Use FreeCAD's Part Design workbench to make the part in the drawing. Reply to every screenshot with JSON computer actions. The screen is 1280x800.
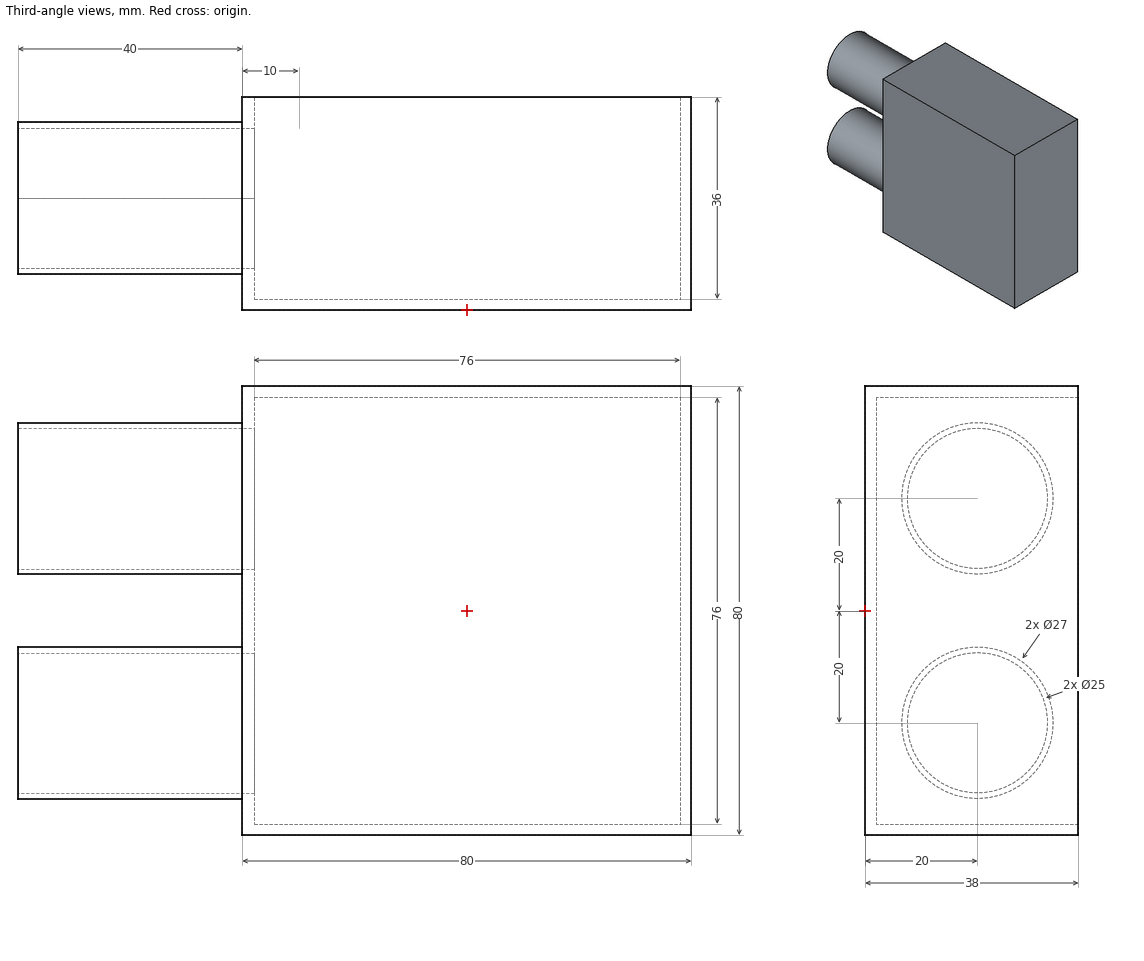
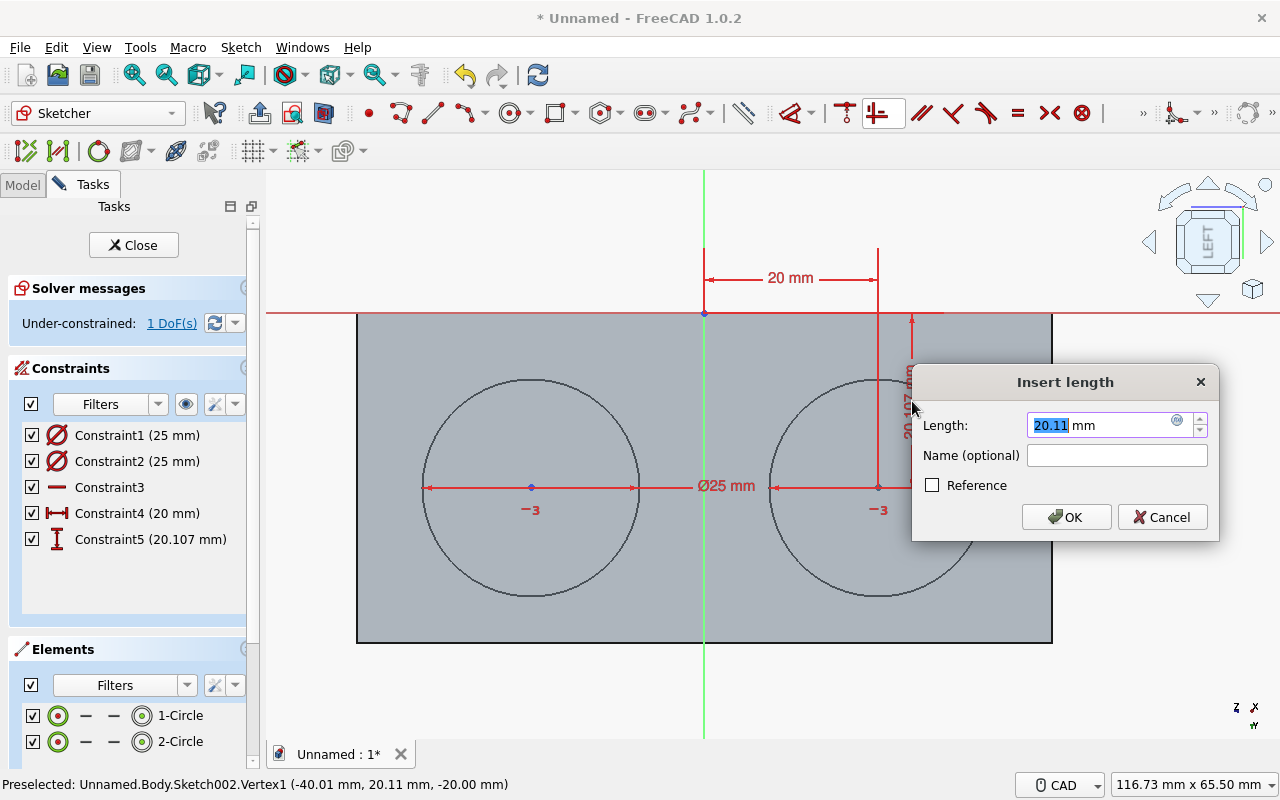
{"action": "type", "text": "20"}
{"action": "key", "text": "Return"}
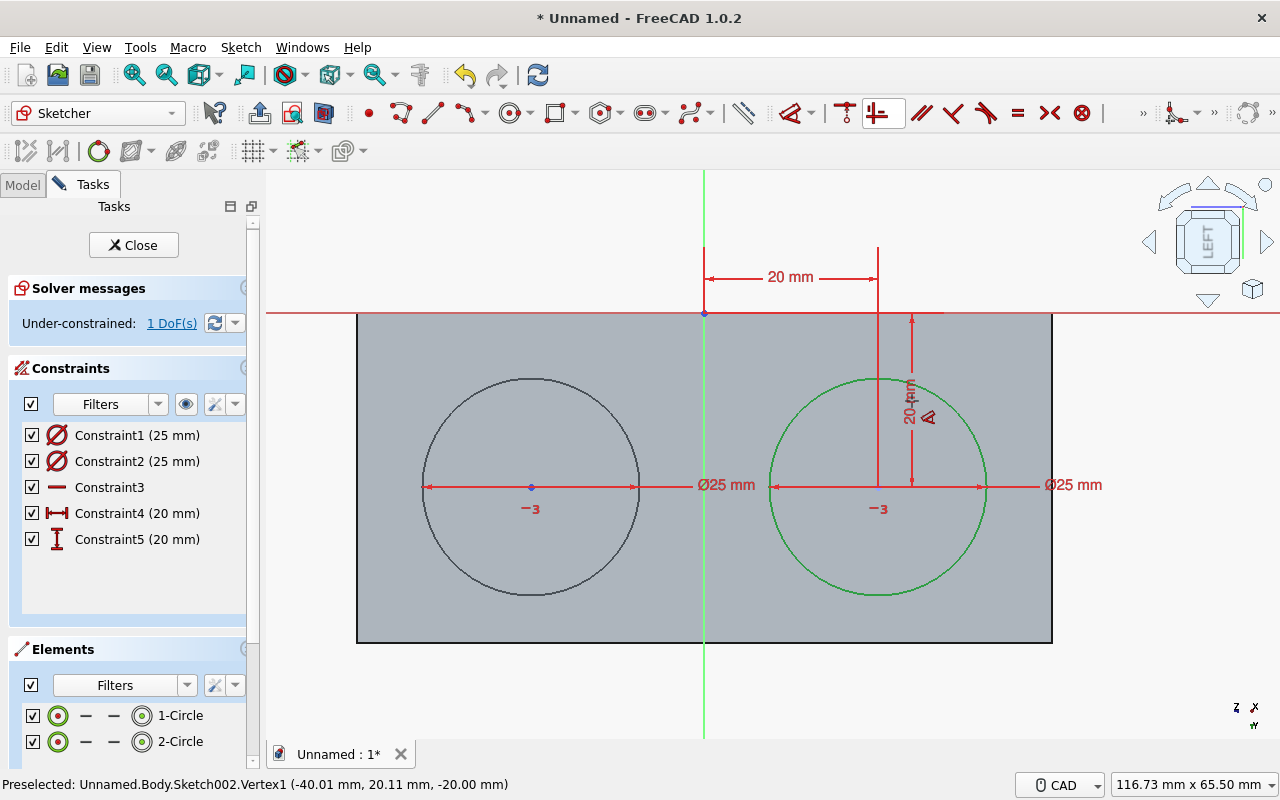
{"action": "left_click", "coordinate": [531, 487]}
{"action": "left_click", "coordinate": [618, 279]}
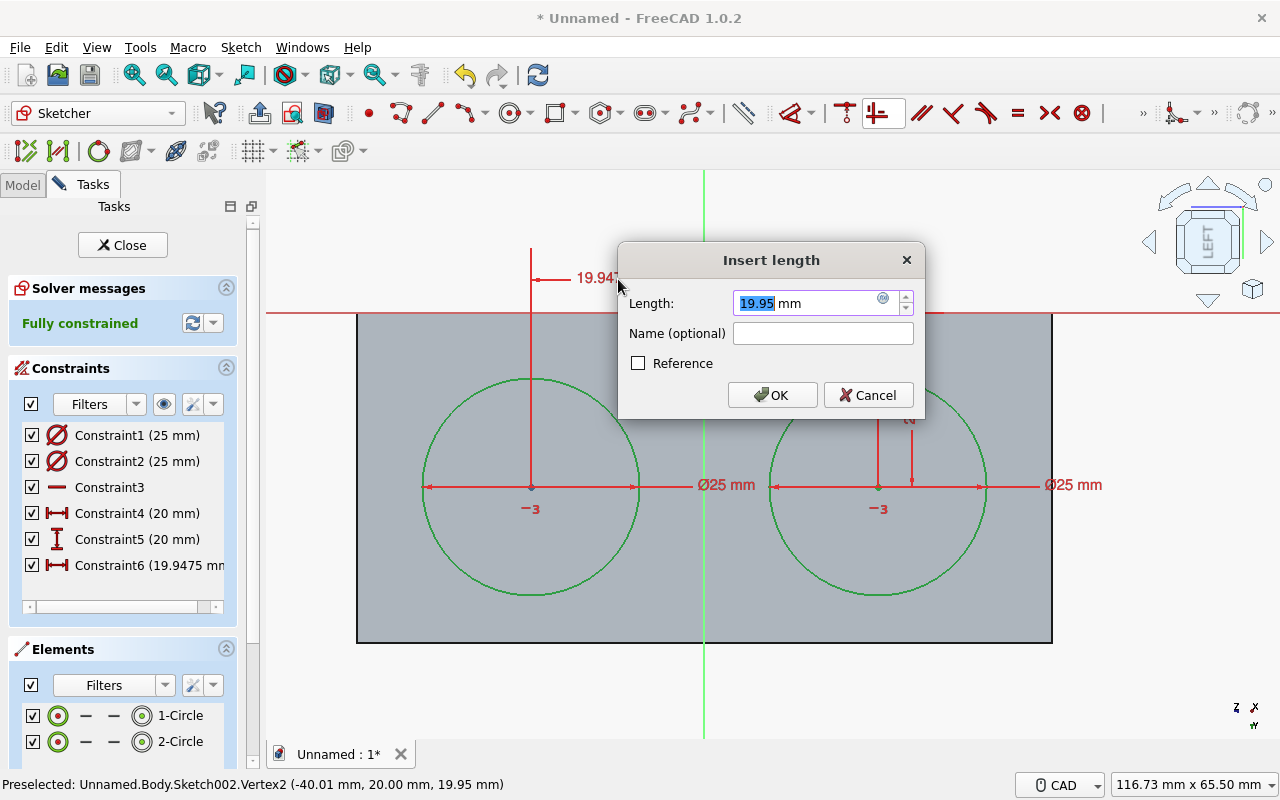
{"action": "type", "text": "20"}
{"action": "key", "text": "Return"}
{"action": "key", "text": "Escape"}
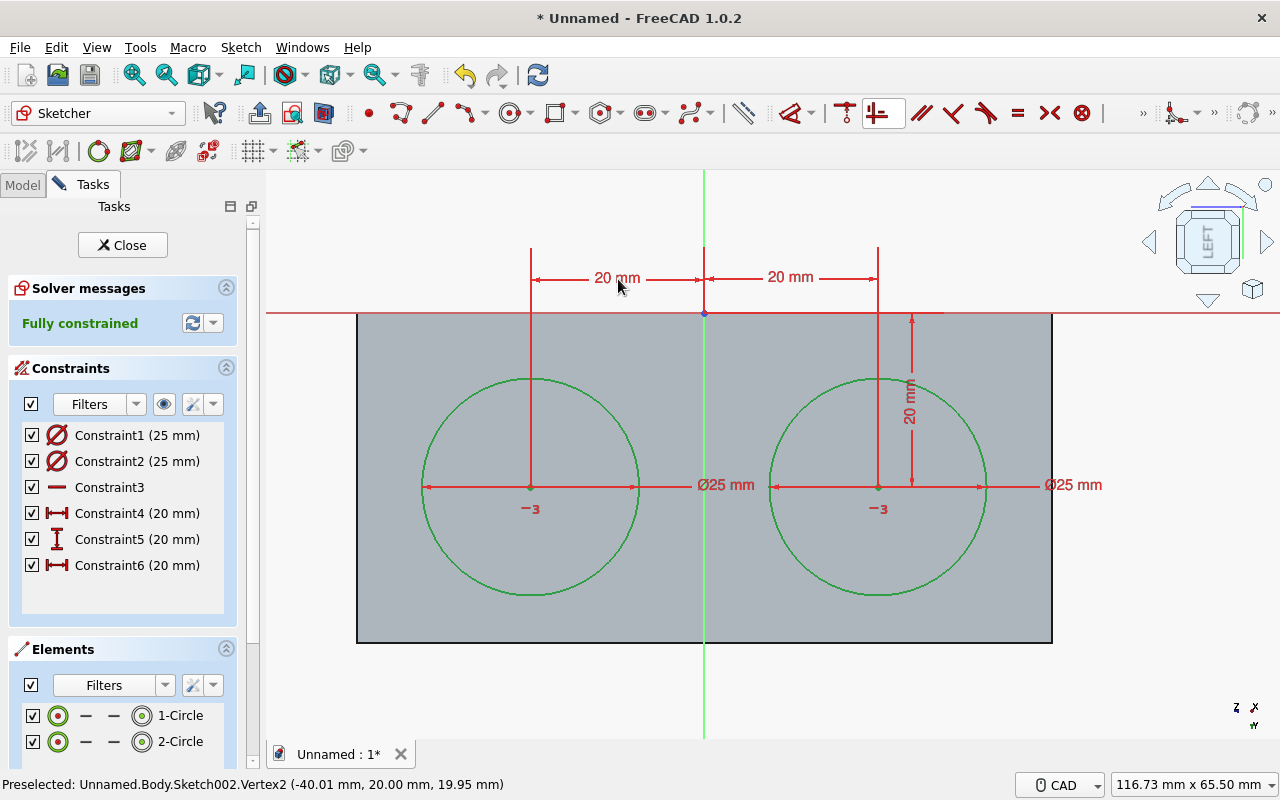
{"action": "left_click", "coordinate": [123, 245]}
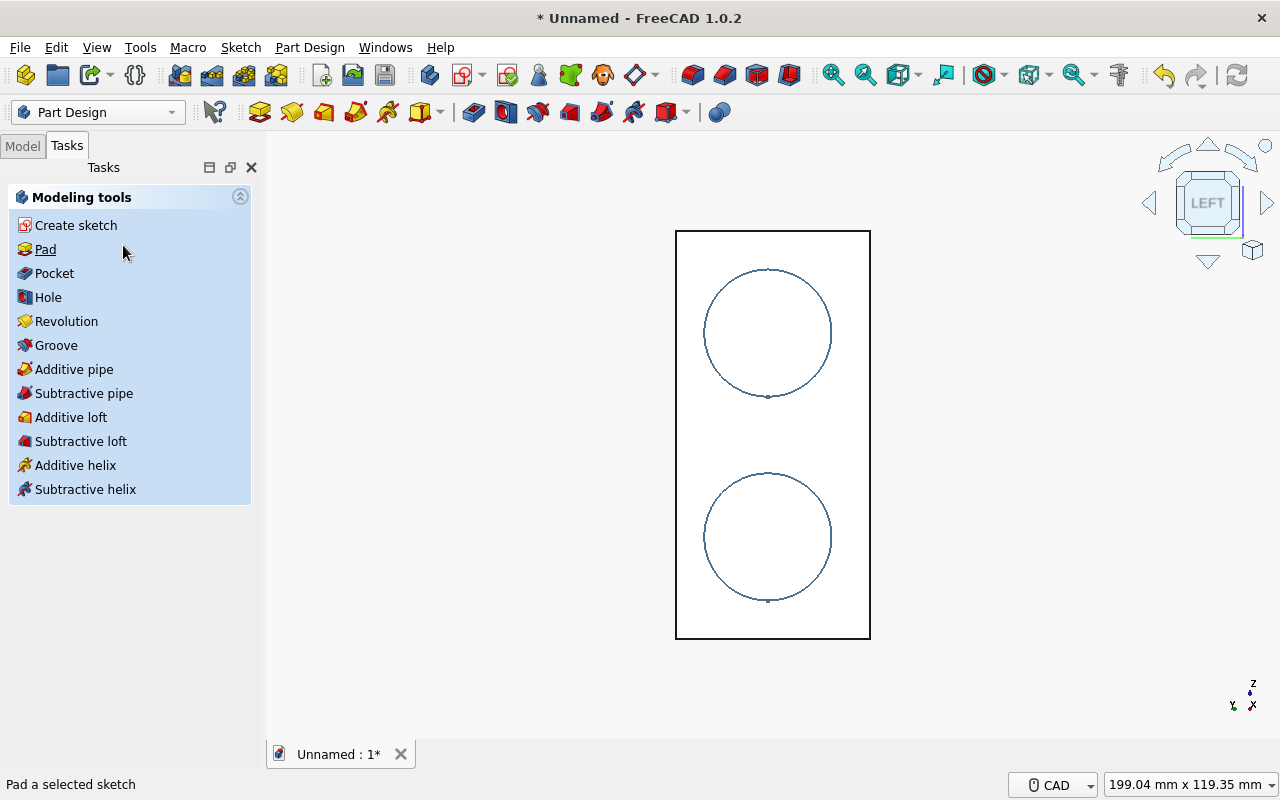
{"action": "left_click", "coordinate": [474, 112]}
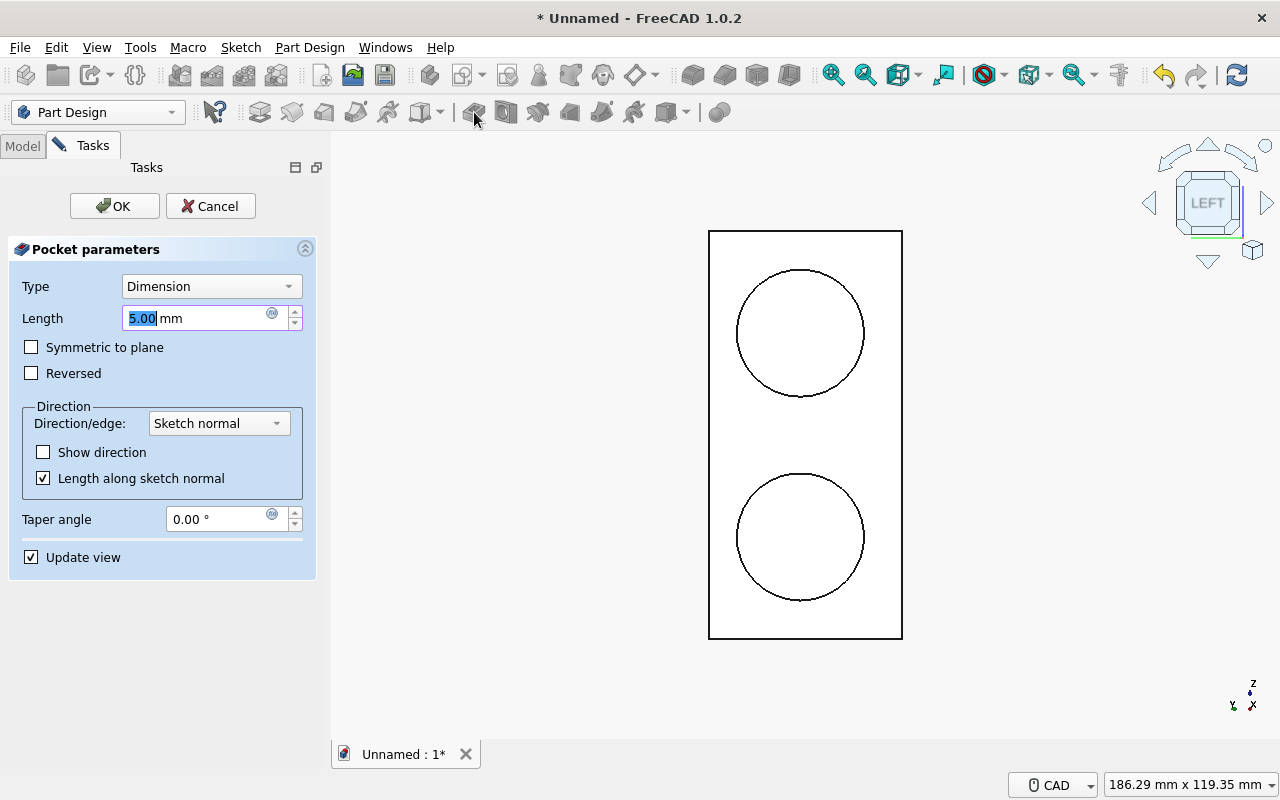
{"action": "type", "text": "10"}
{"action": "key", "text": "Tab"}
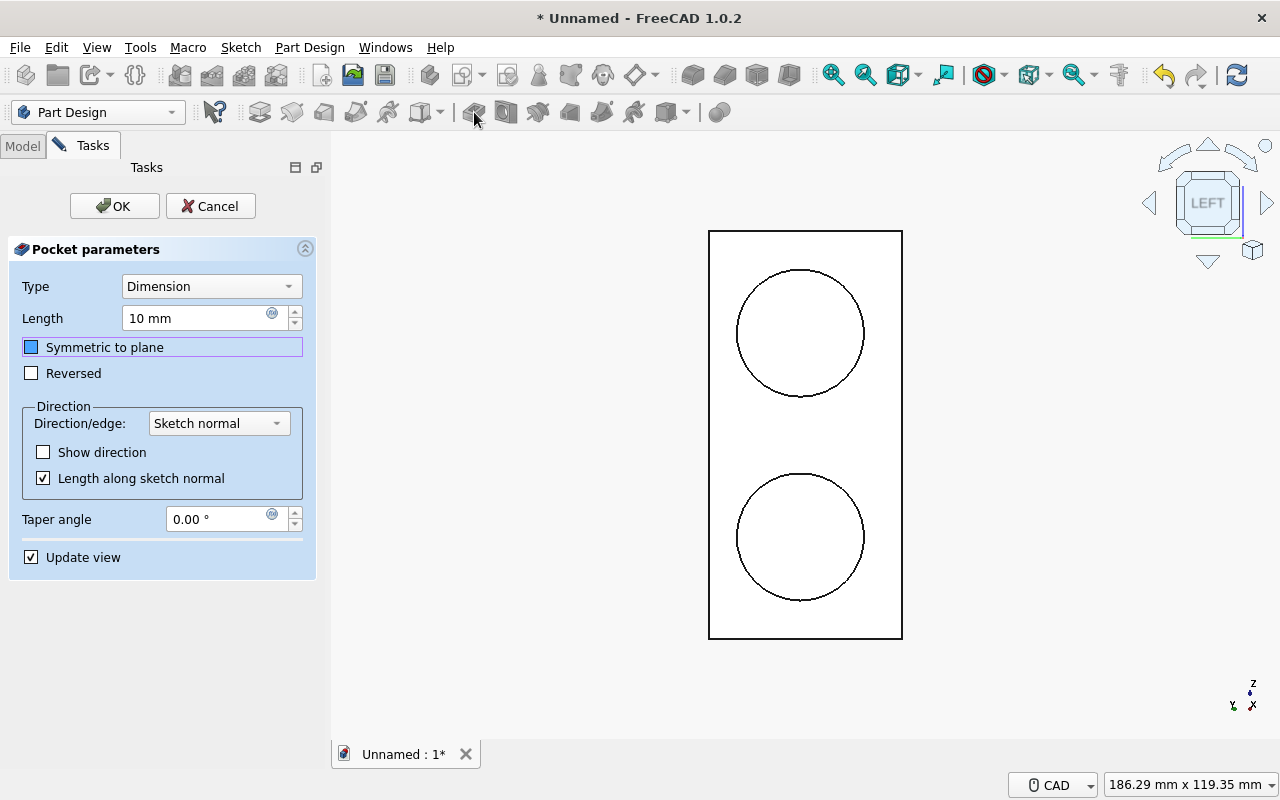
{"action": "left_click", "coordinate": [115, 206]}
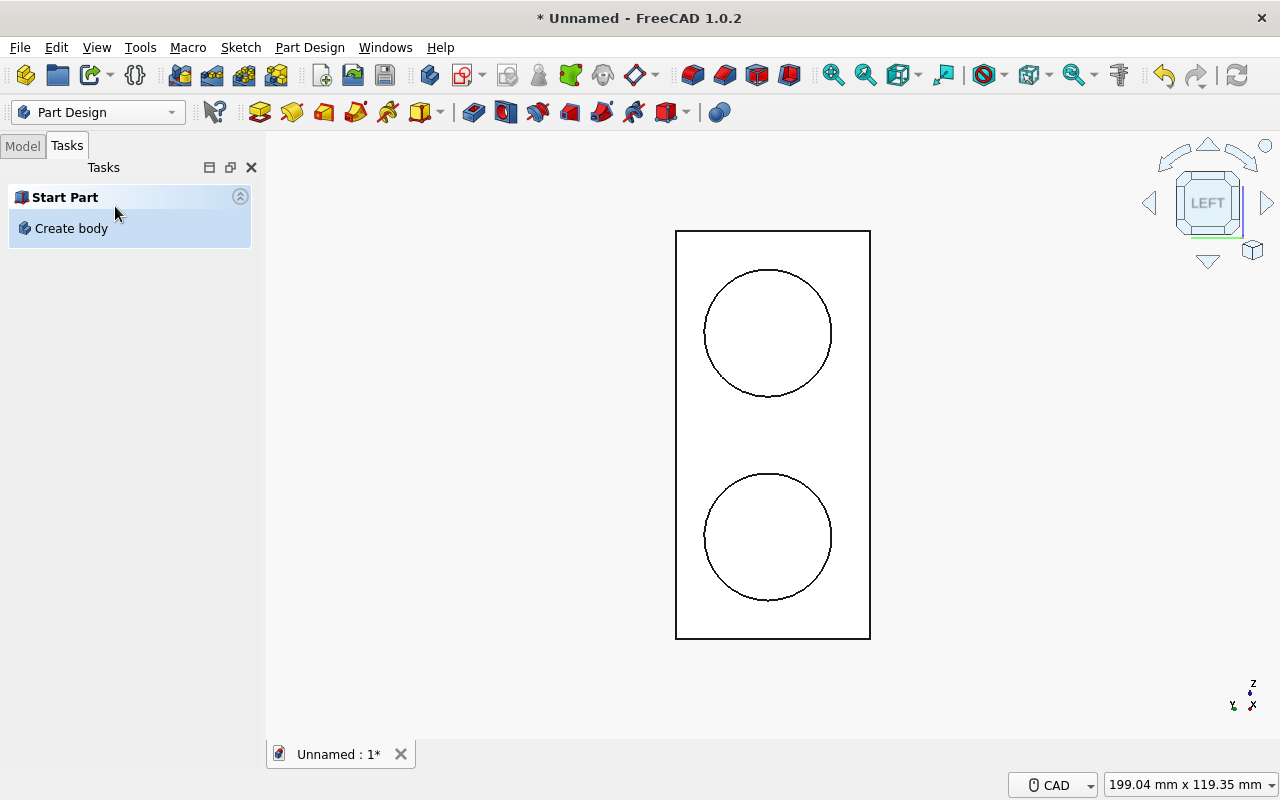
{"action": "left_click", "coordinate": [23, 145]}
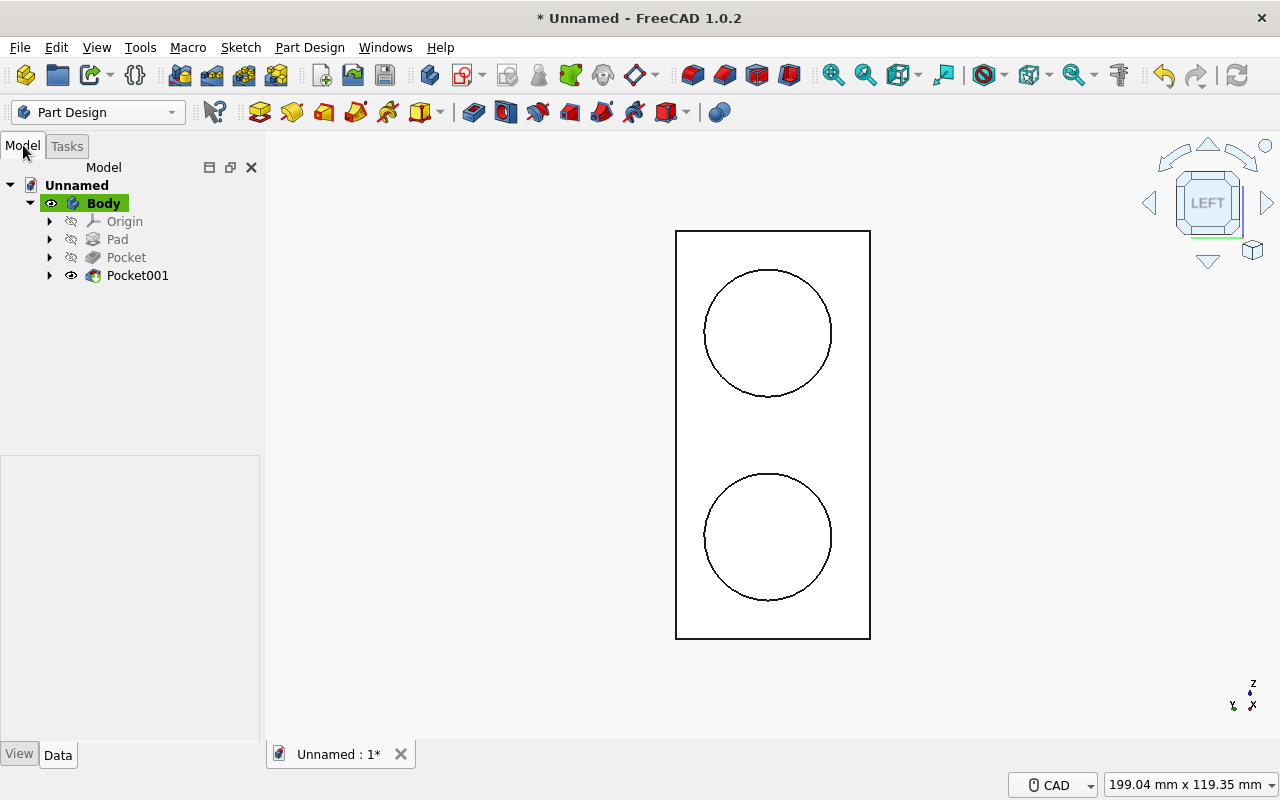
{"action": "left_click", "coordinate": [50, 221]}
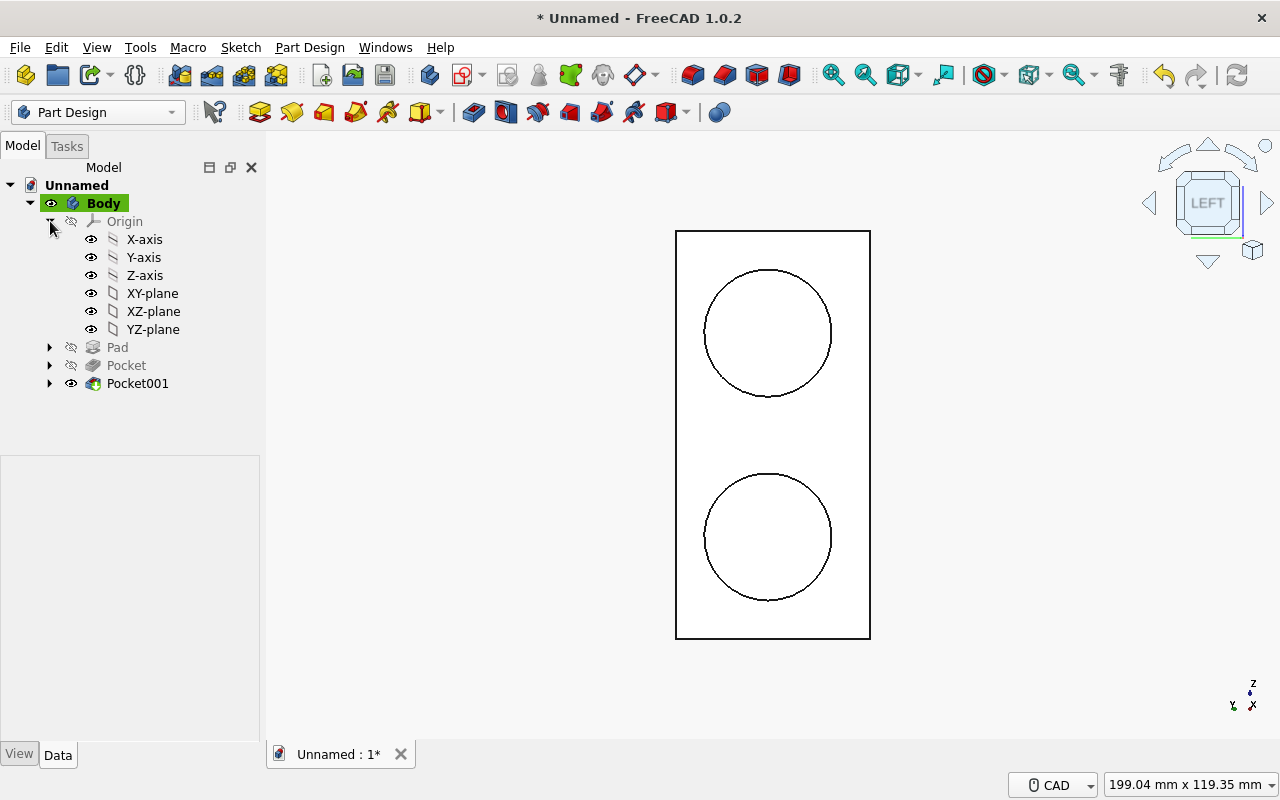
{"action": "left_click", "coordinate": [136, 329]}